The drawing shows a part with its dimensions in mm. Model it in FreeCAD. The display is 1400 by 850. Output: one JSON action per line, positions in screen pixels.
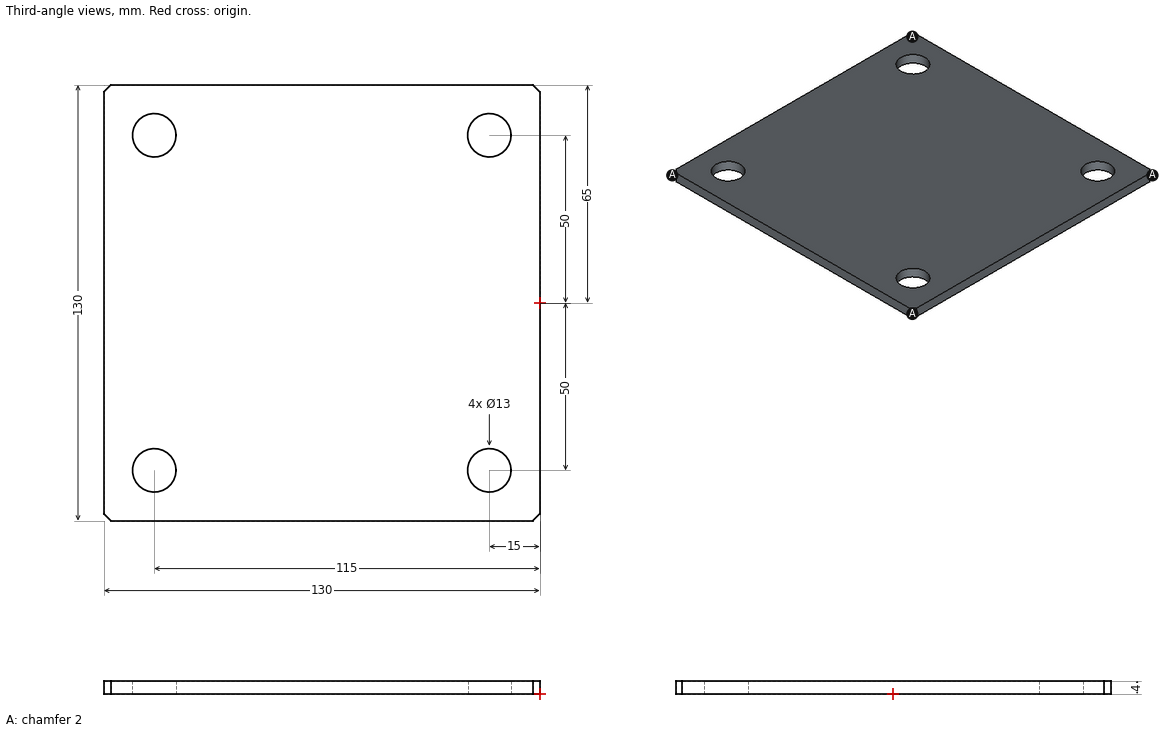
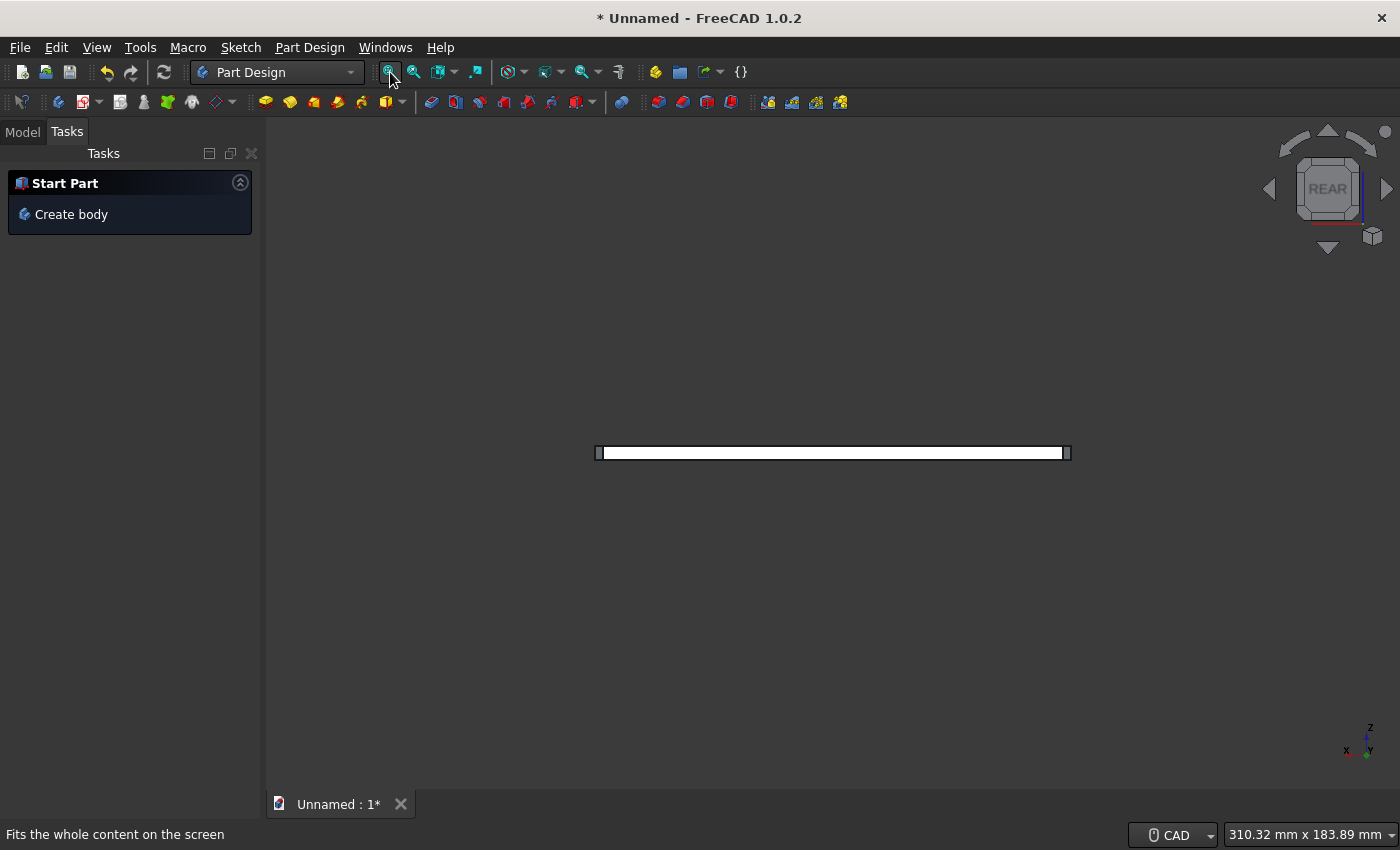
{"action": "key", "text": "5"}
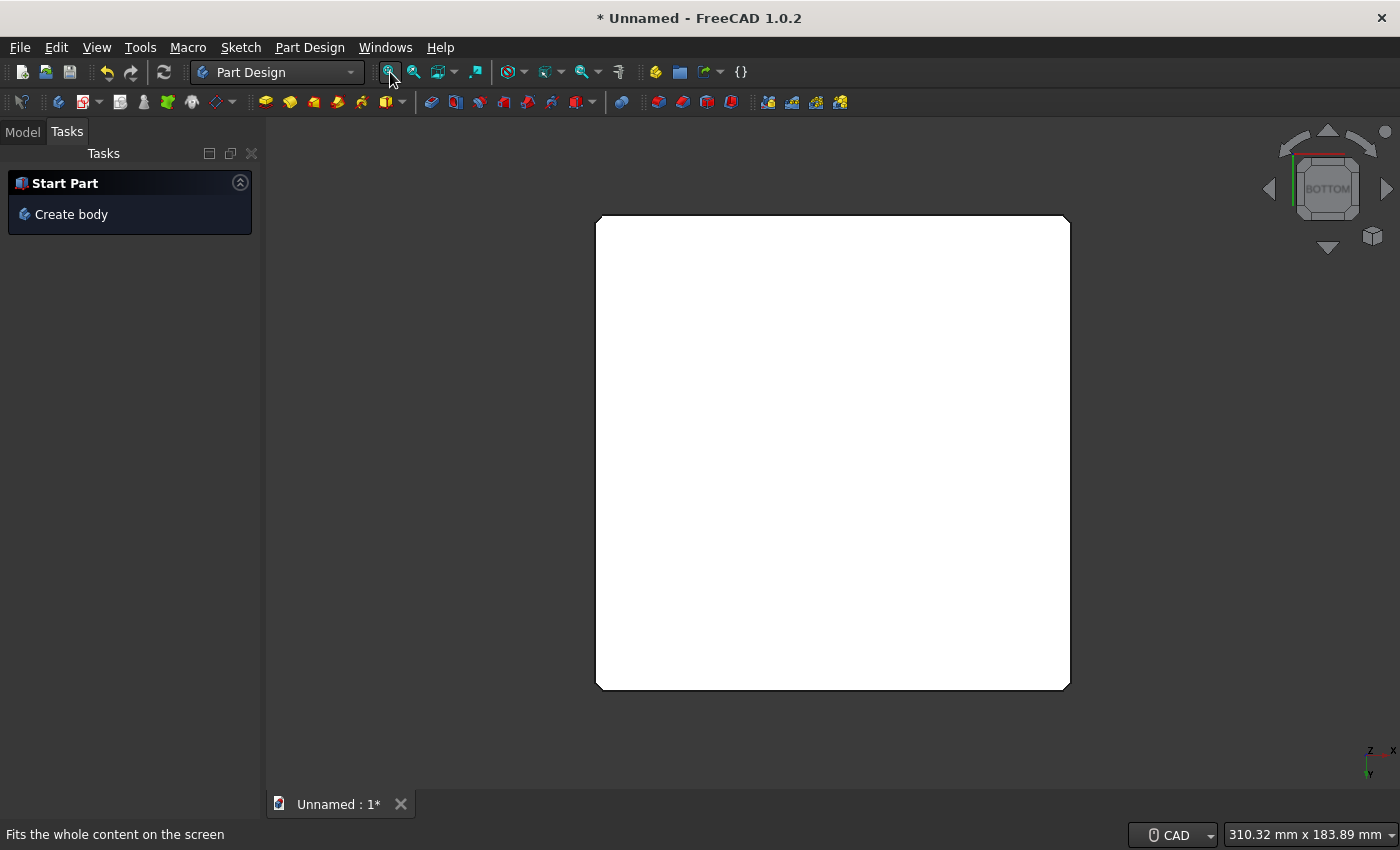
{"action": "left_click", "coordinate": [833, 452]}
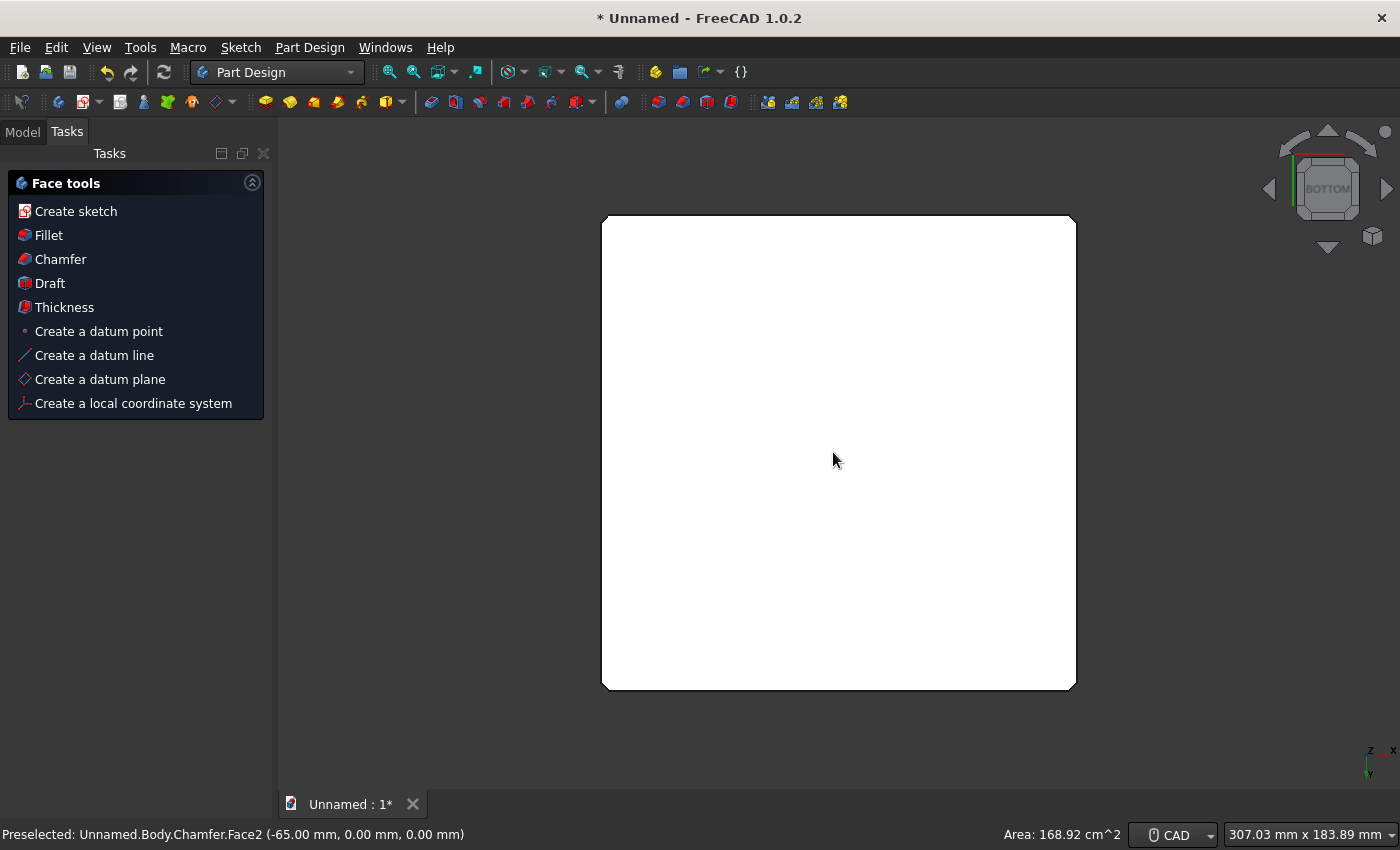
{"action": "left_click", "coordinate": [84, 102]}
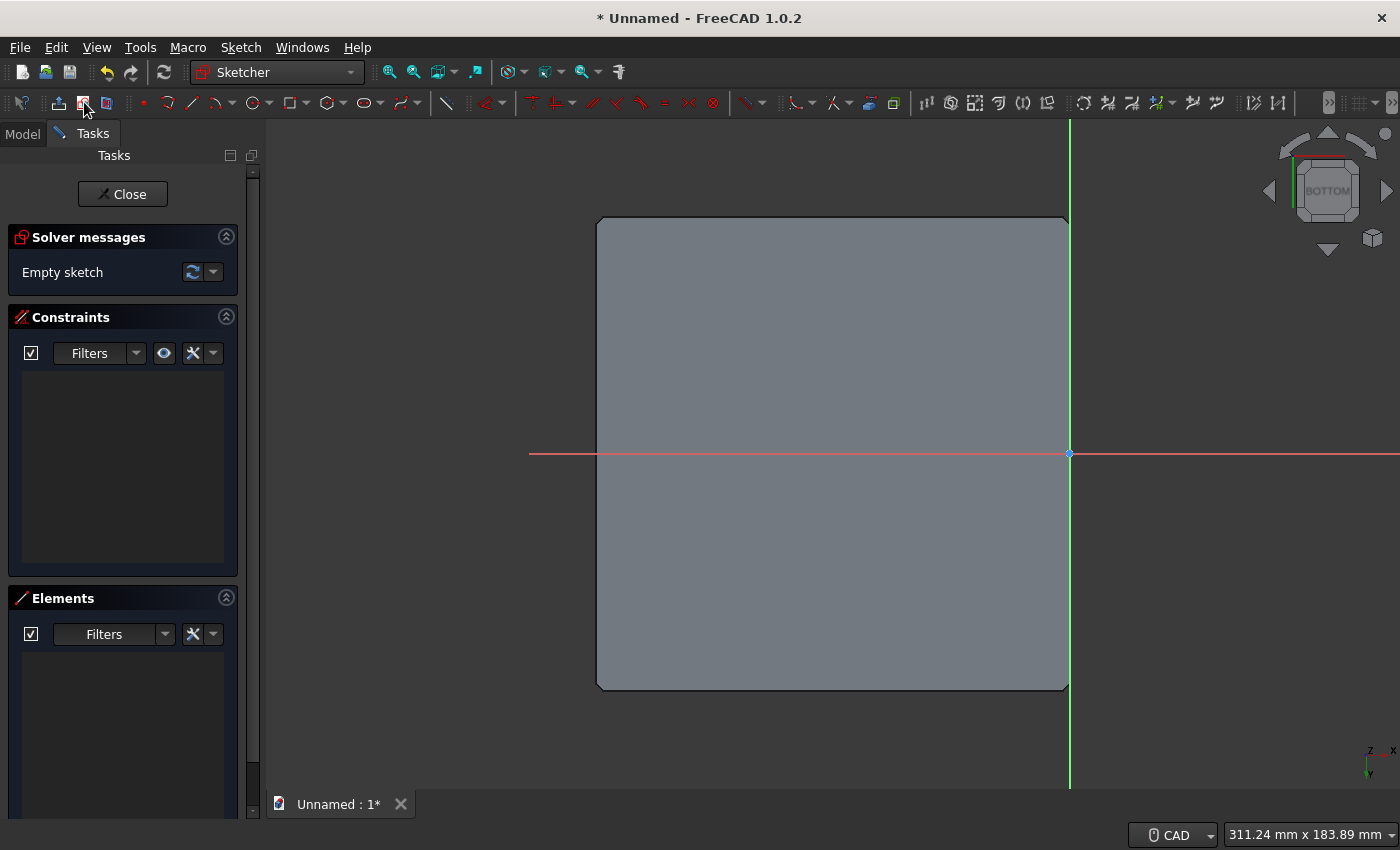
{"action": "left_click", "coordinate": [254, 104]}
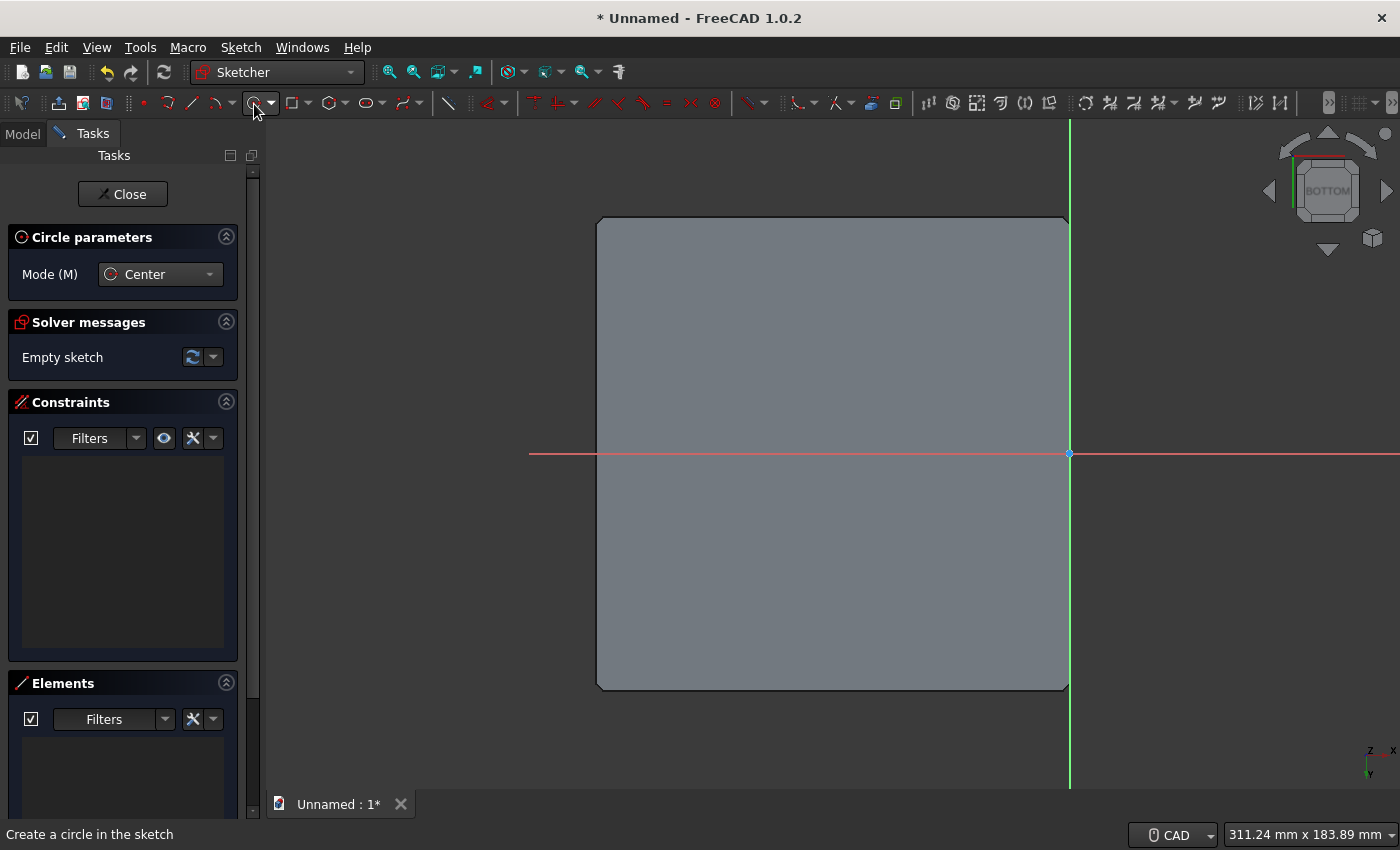
{"action": "left_click", "coordinate": [1015, 272]}
{"action": "mouse_move", "coordinate": [1032, 255]}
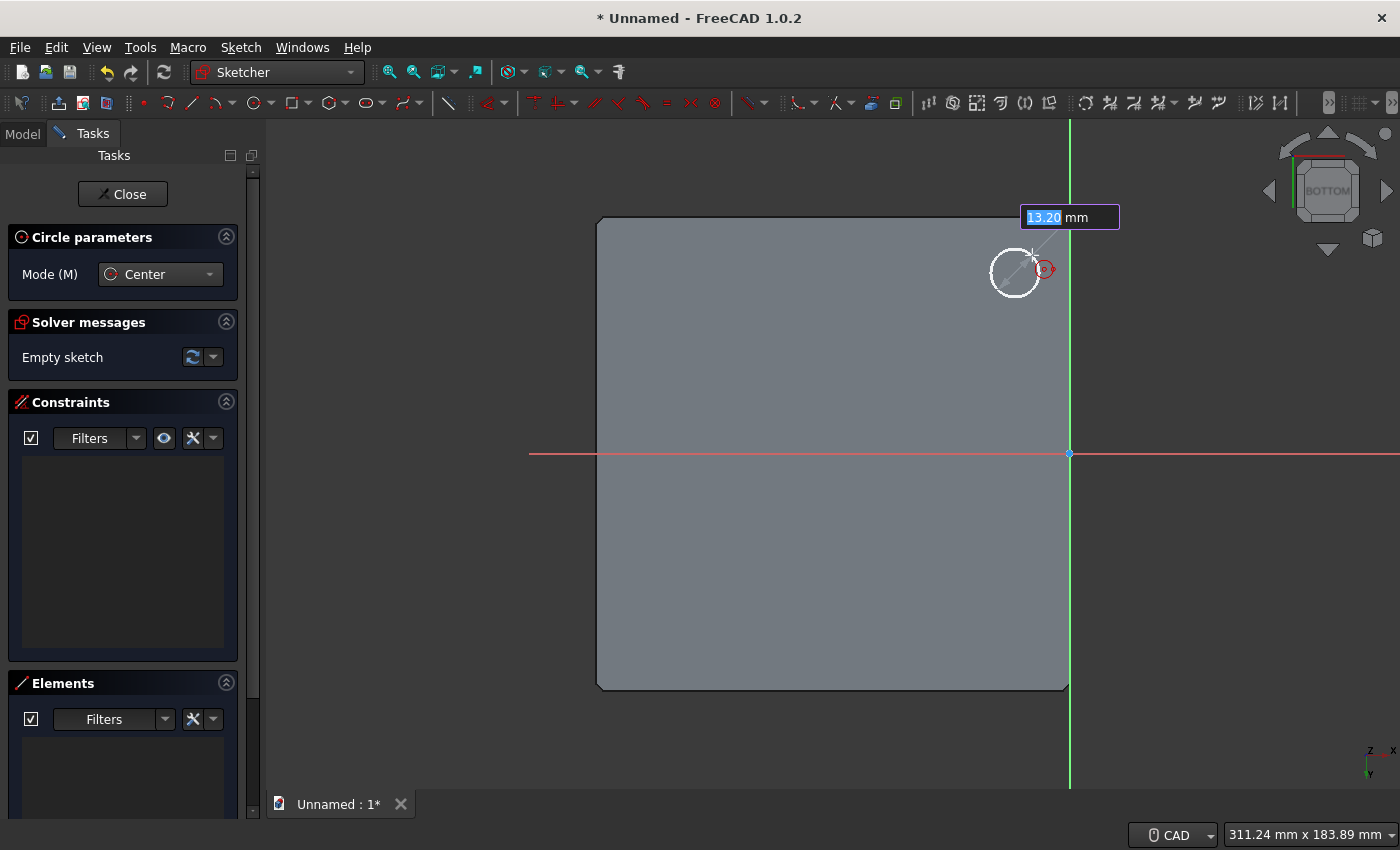
{"action": "type", "text": "13"}
{"action": "key", "text": "Return"}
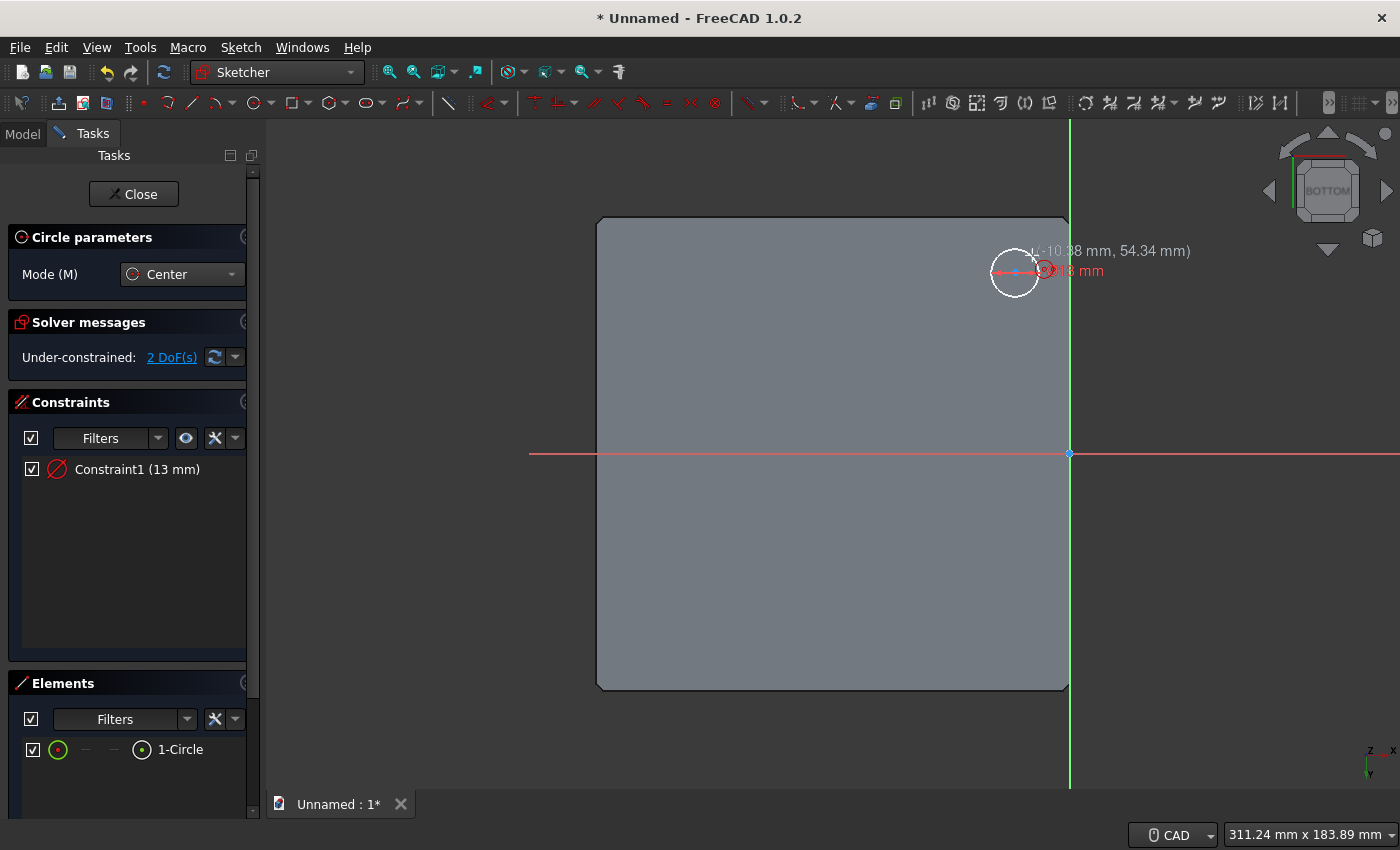
{"action": "left_click", "coordinate": [1015, 636]}
{"action": "mouse_move", "coordinate": [1032, 619]}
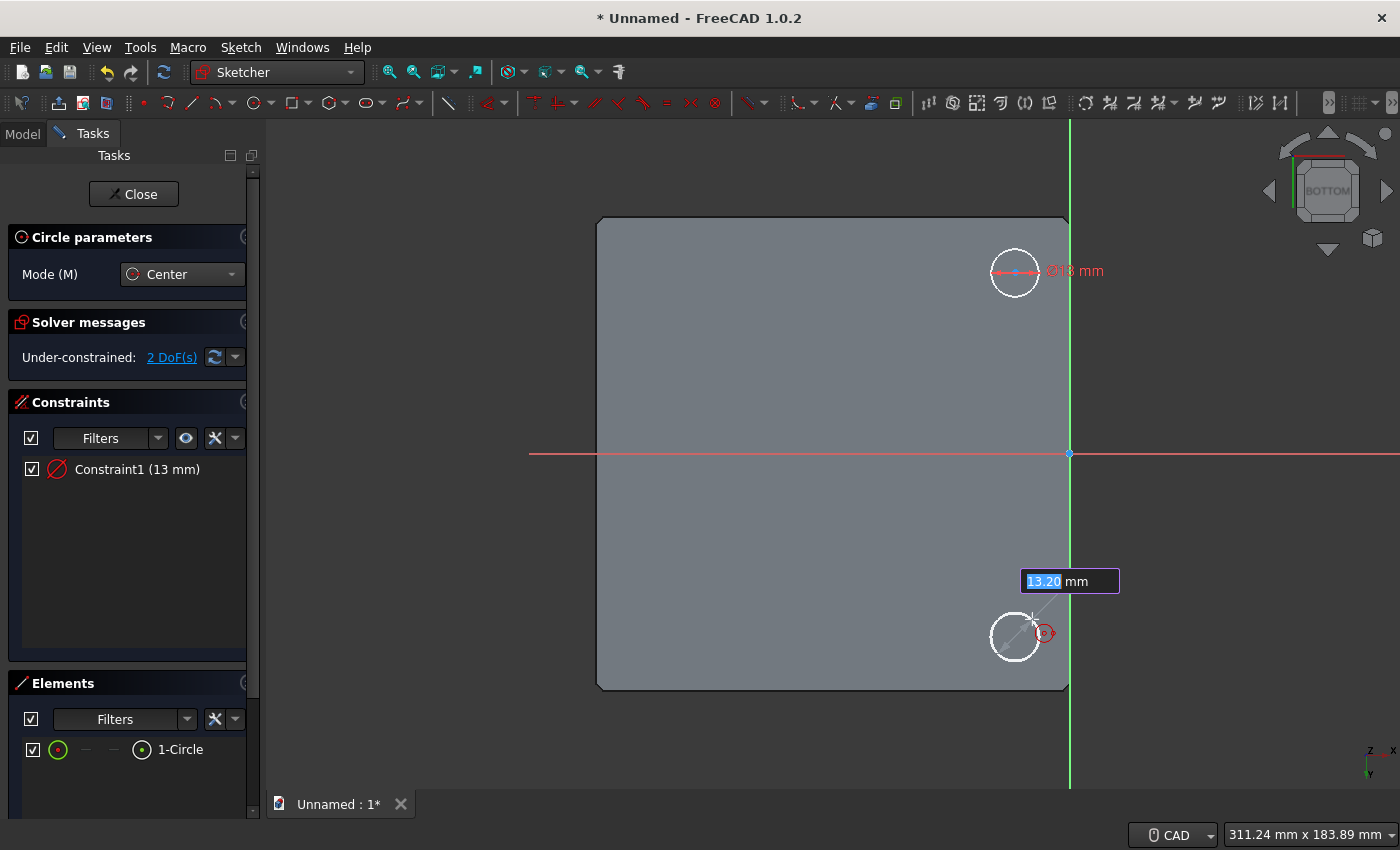
{"action": "type", "text": "13"}
{"action": "key", "text": "Return"}